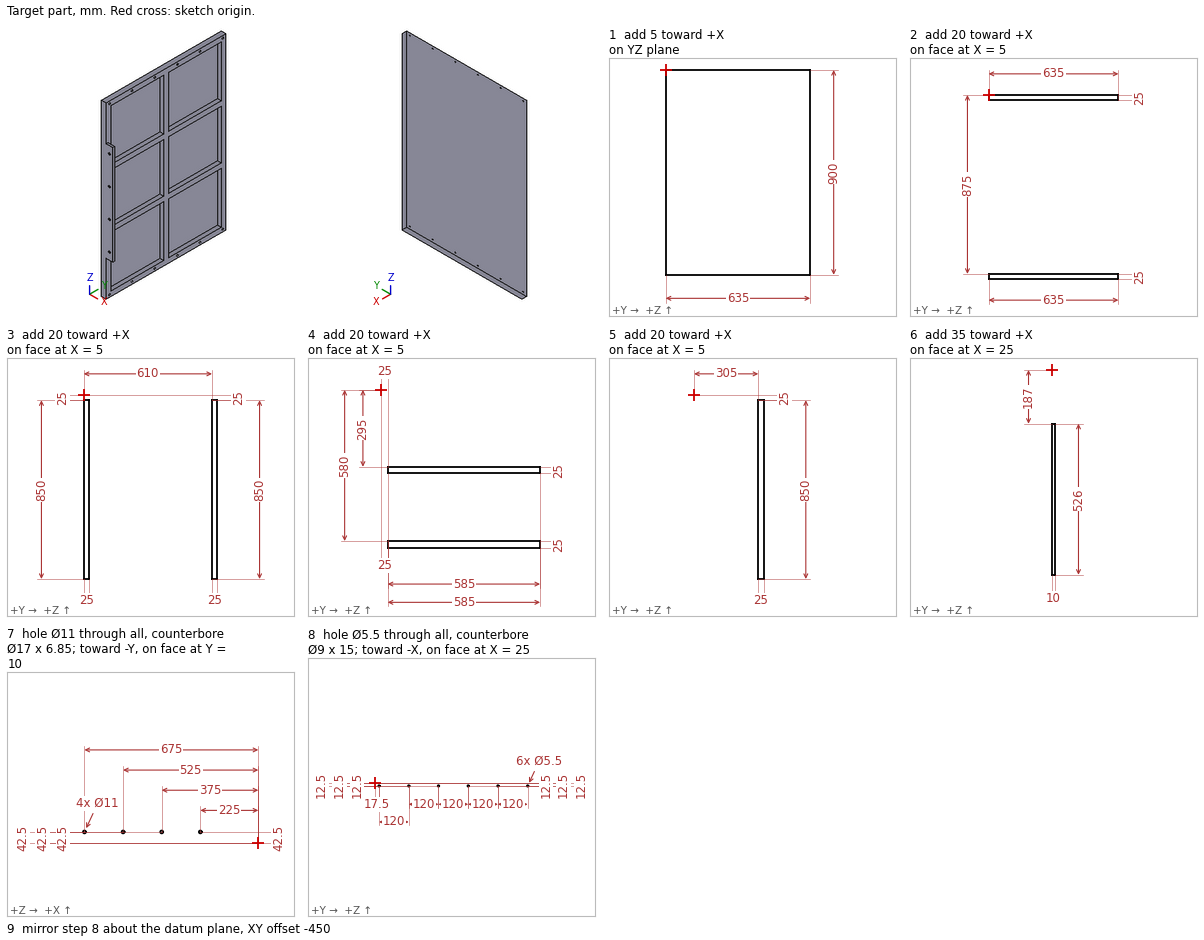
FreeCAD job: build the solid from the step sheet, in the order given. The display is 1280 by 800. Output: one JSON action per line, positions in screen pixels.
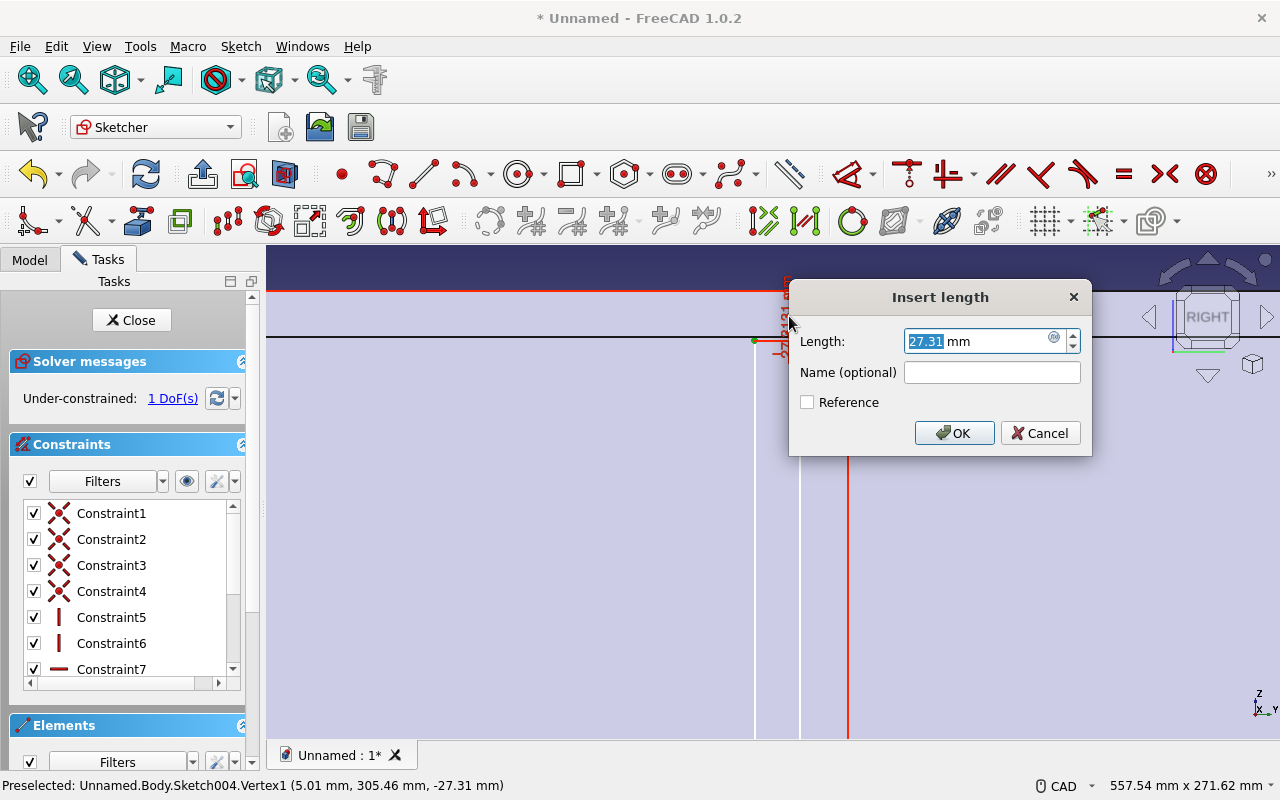
{"action": "type", "text": "25"}
{"action": "key", "text": "Return"}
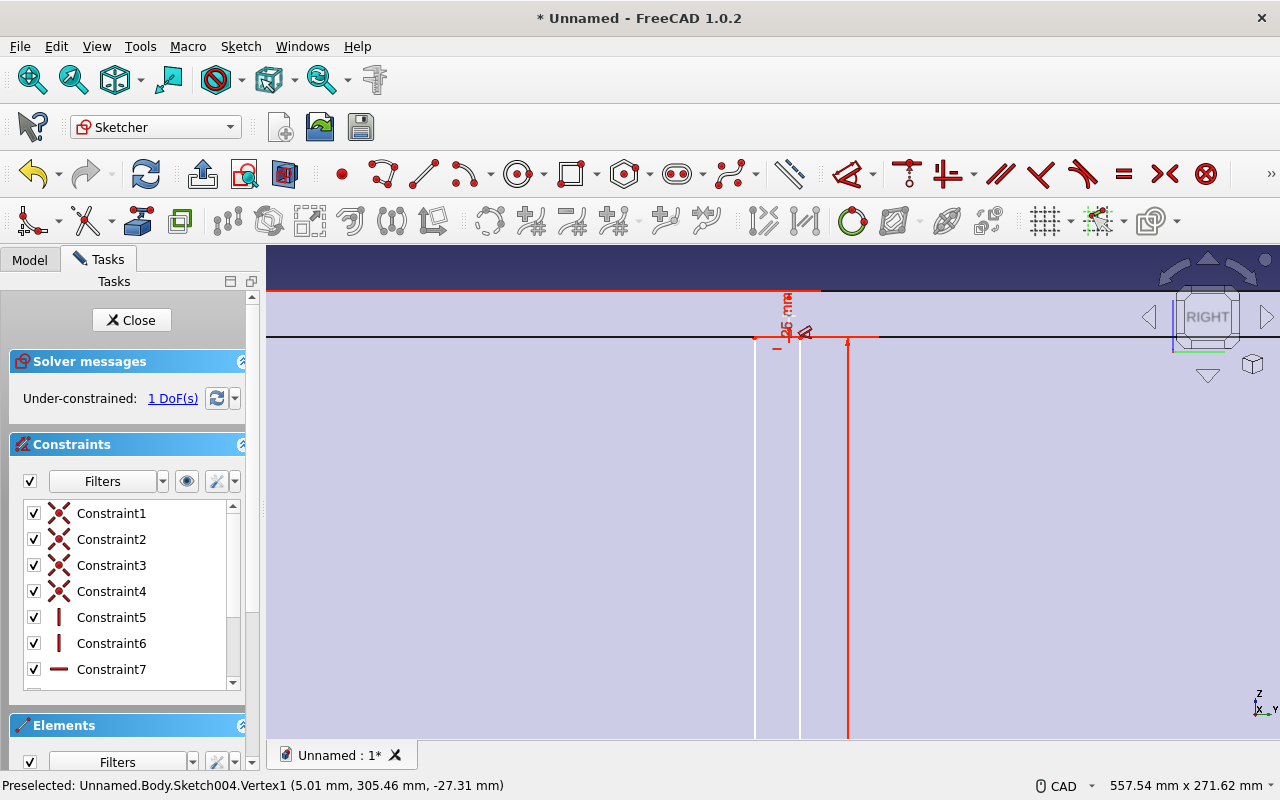
{"action": "scroll", "coordinate": [756, 342], "scroll_direction": "down", "scroll_amount": 8}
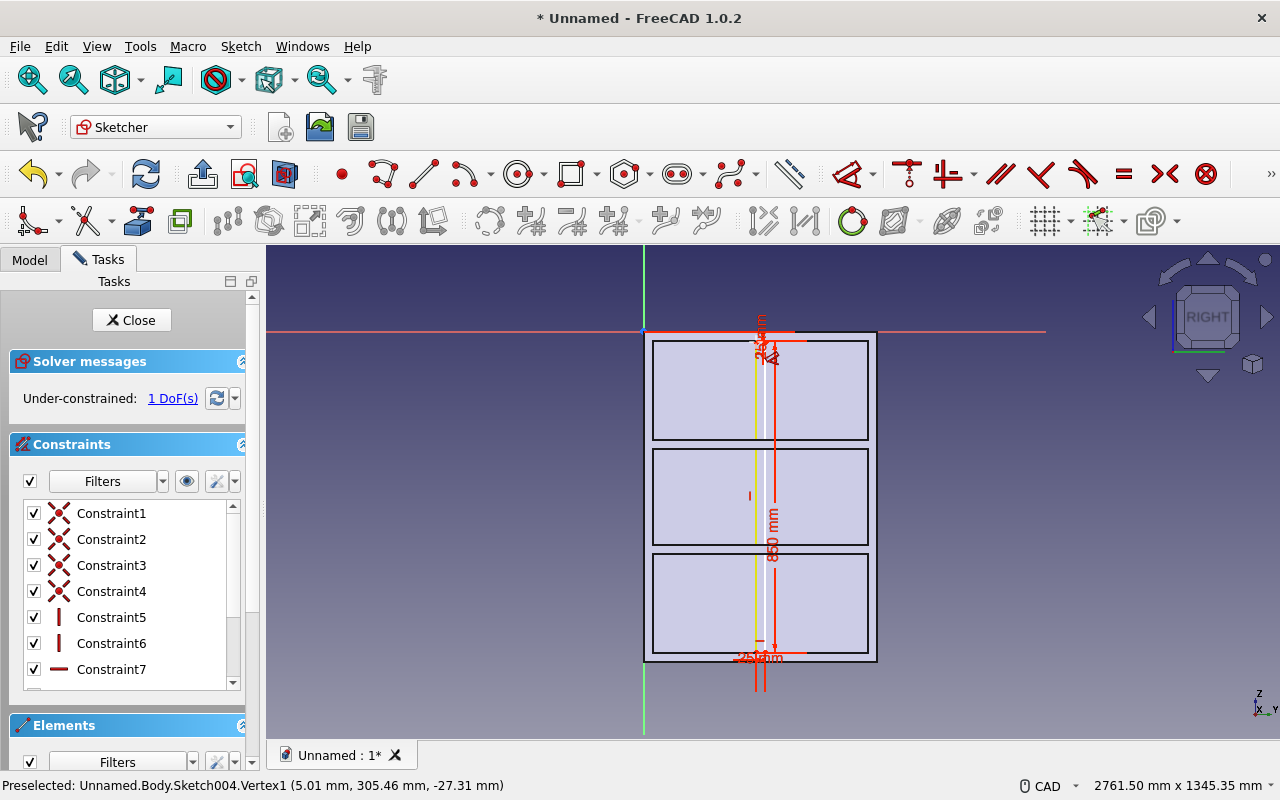
{"action": "scroll", "coordinate": [756, 341], "scroll_direction": "up", "scroll_amount": 2}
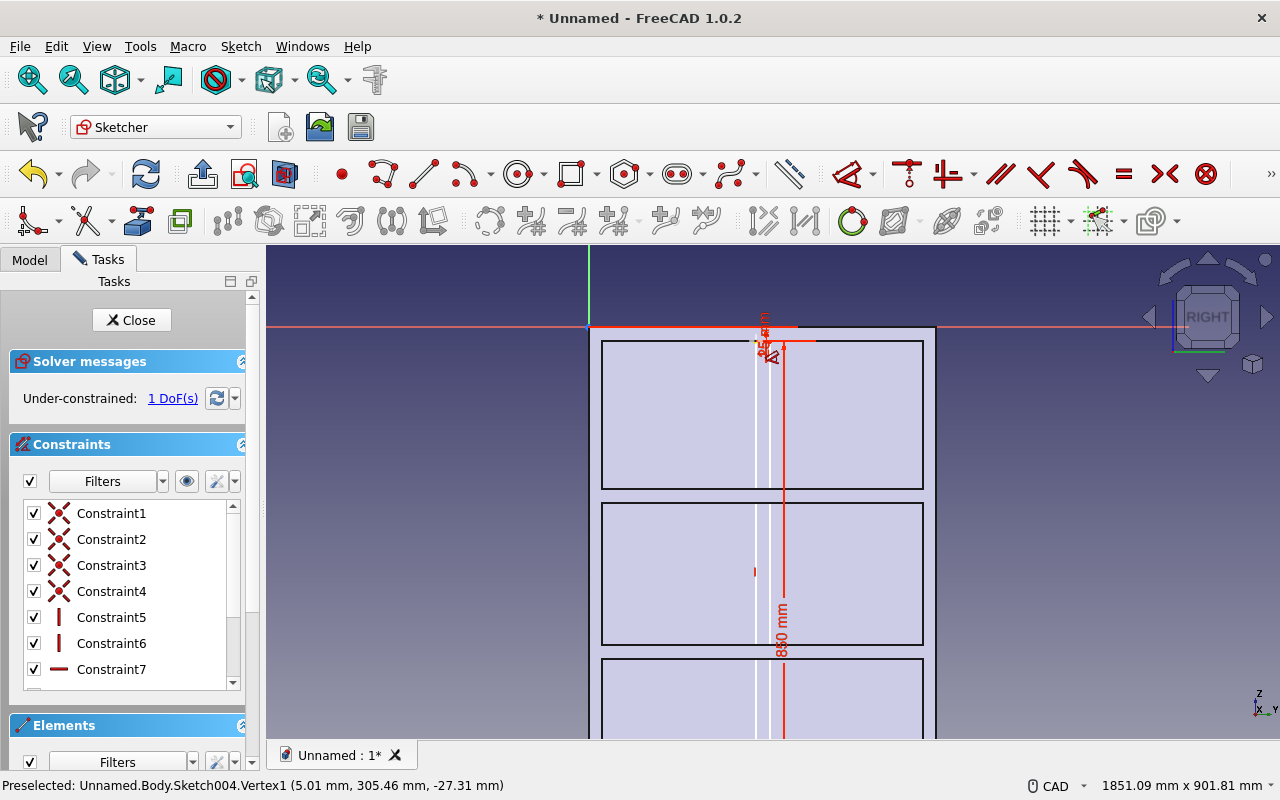
{"action": "left_click", "coordinate": [756, 341]}
{"action": "left_click", "coordinate": [672, 293]}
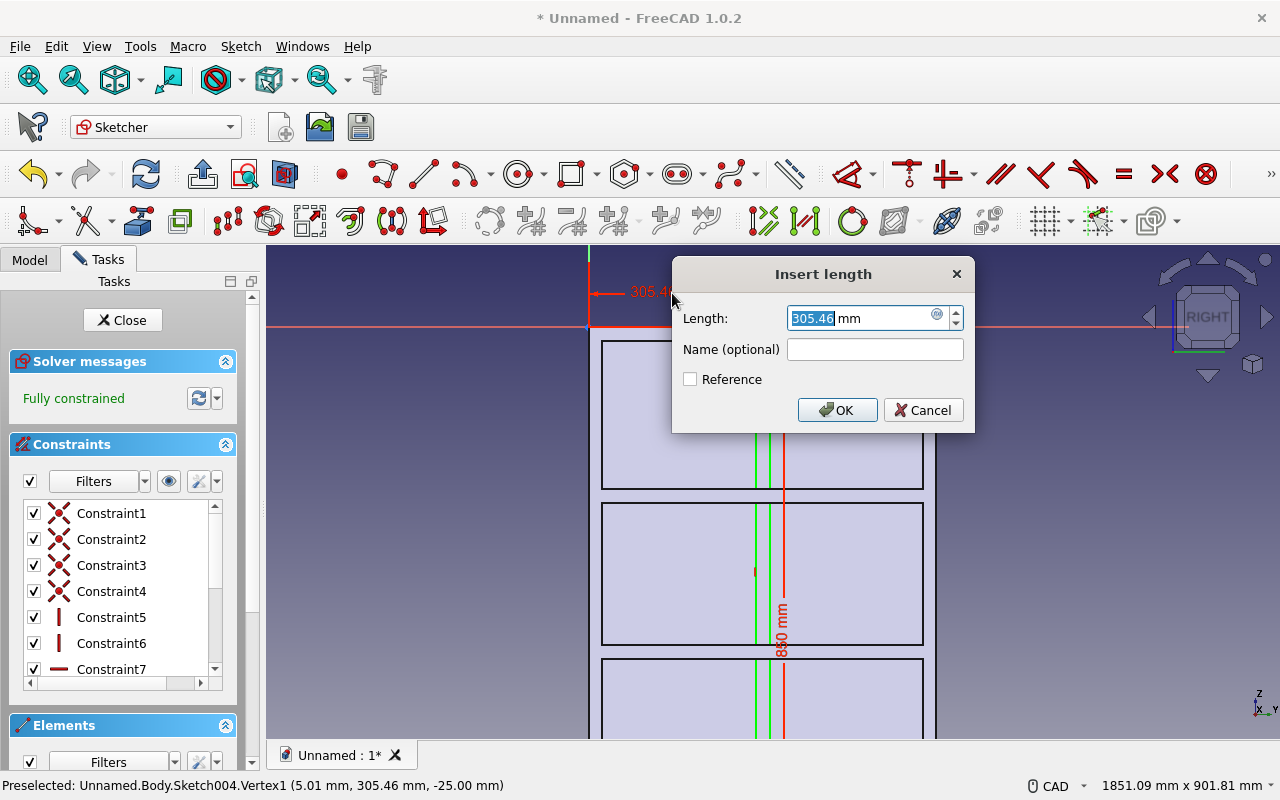
{"action": "type", "text": "305"}
{"action": "key", "text": "Return"}
{"action": "key", "text": "Escape"}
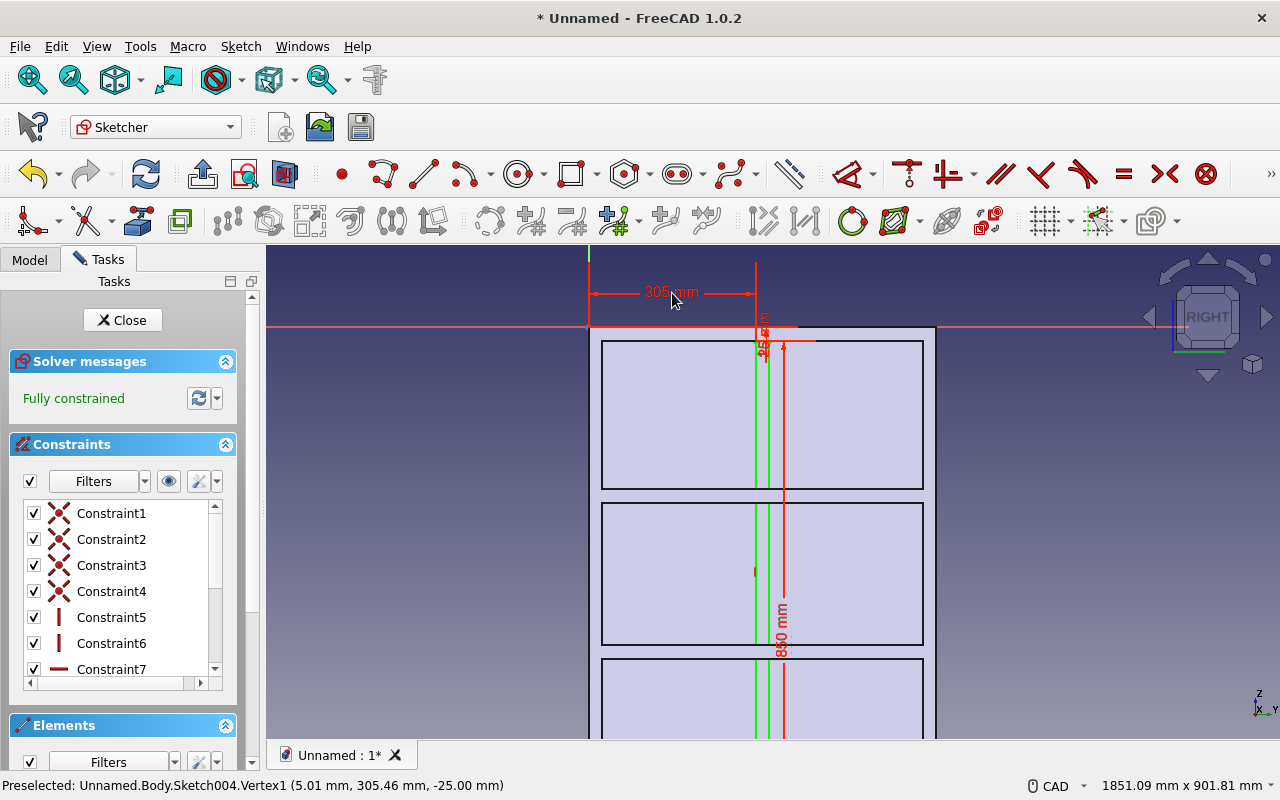
{"action": "left_click", "coordinate": [123, 320]}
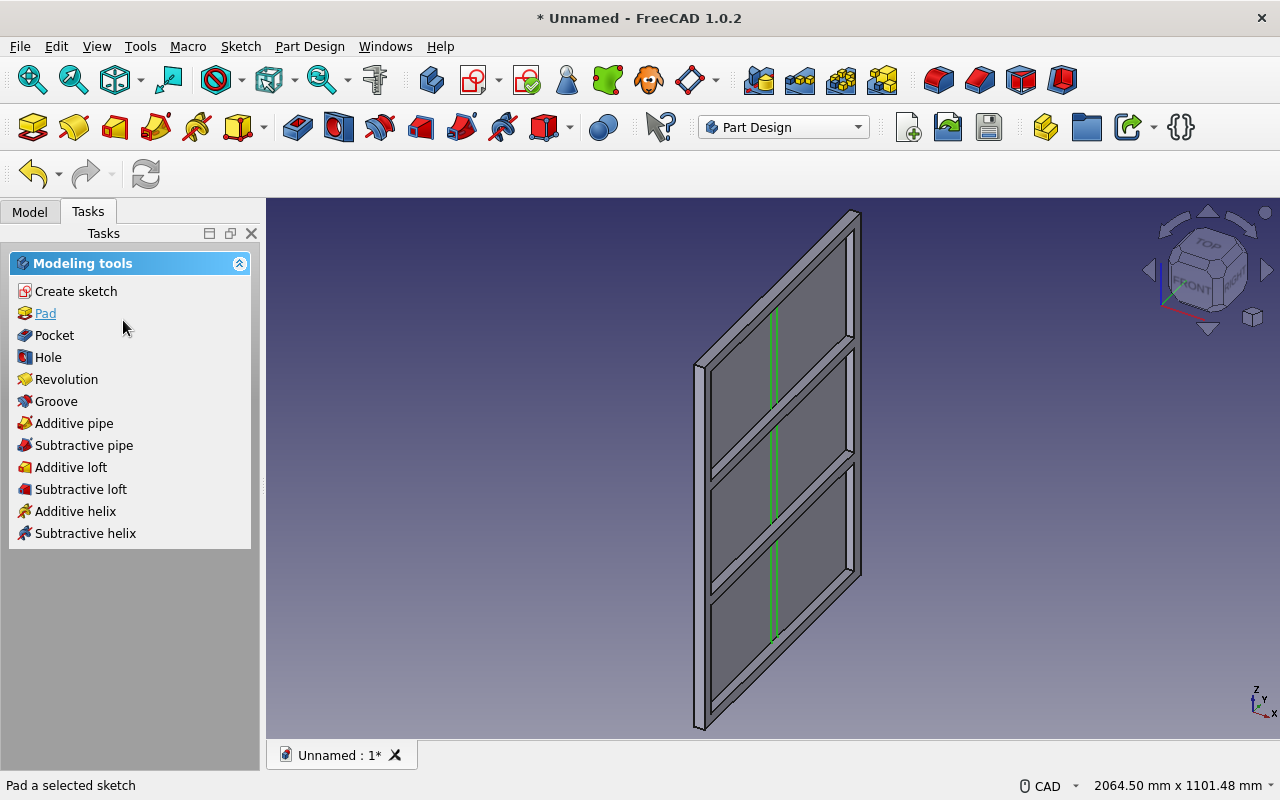
{"action": "left_click", "coordinate": [33, 128]}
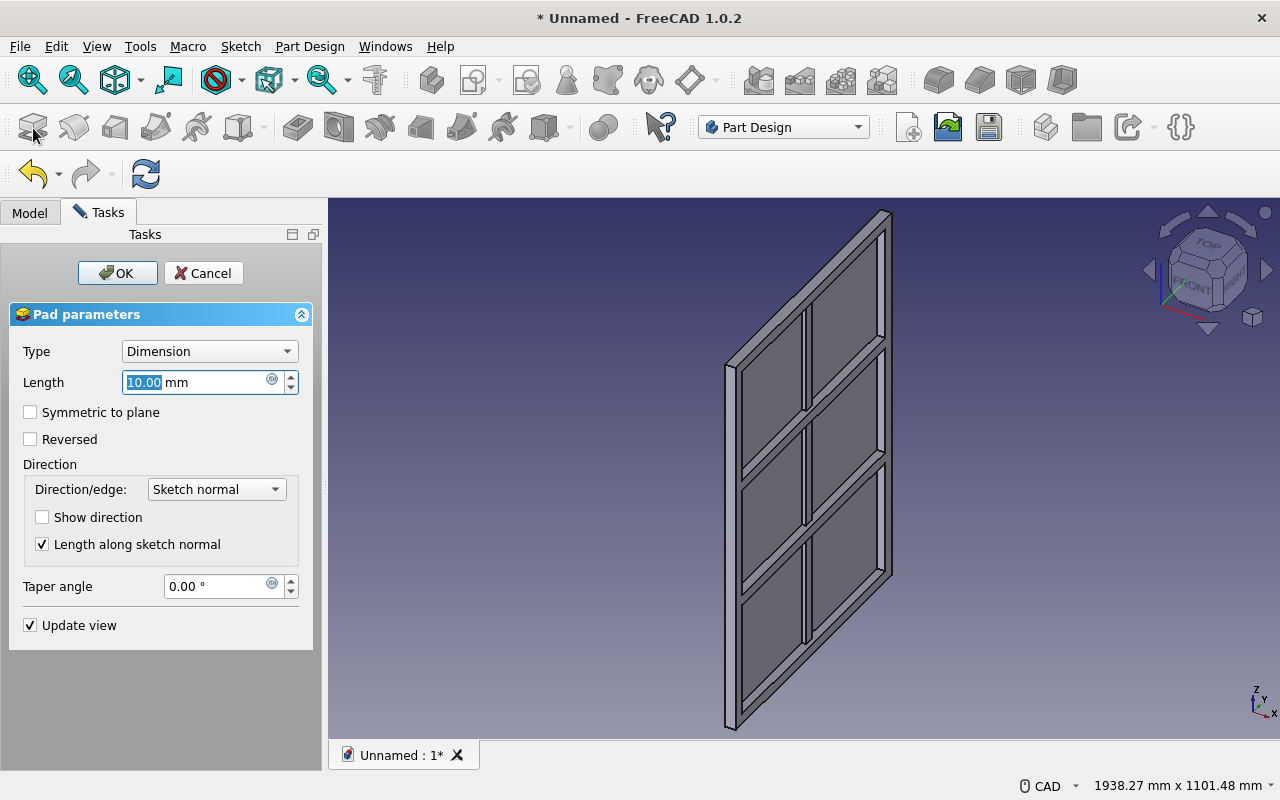
{"action": "type", "text": "20"}
{"action": "key", "text": "Tab"}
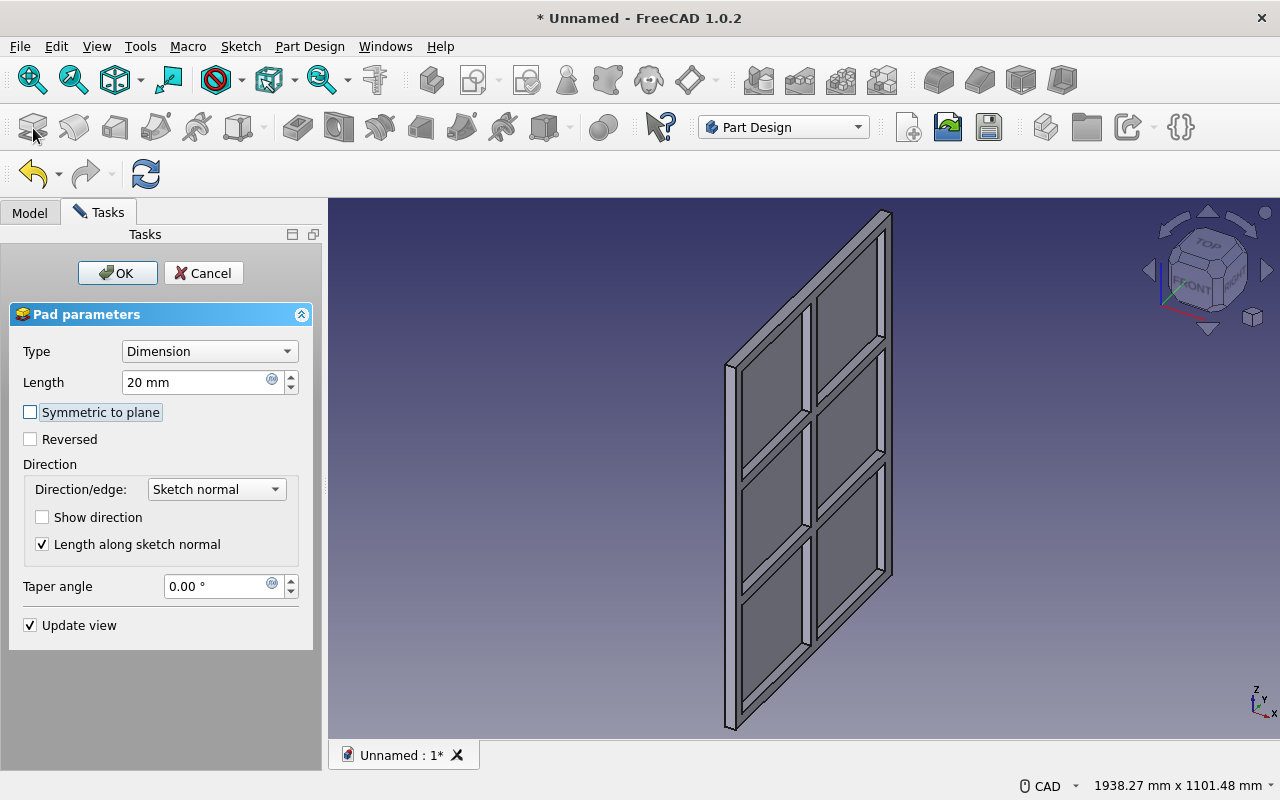
{"action": "left_click", "coordinate": [118, 273]}